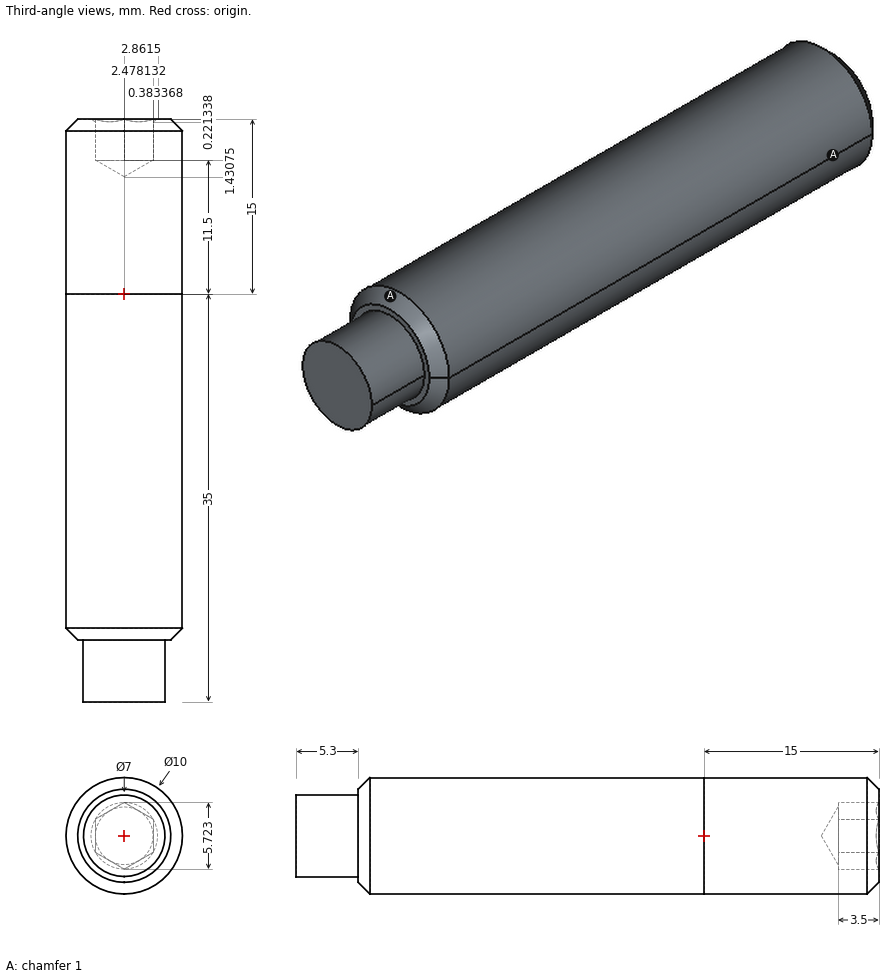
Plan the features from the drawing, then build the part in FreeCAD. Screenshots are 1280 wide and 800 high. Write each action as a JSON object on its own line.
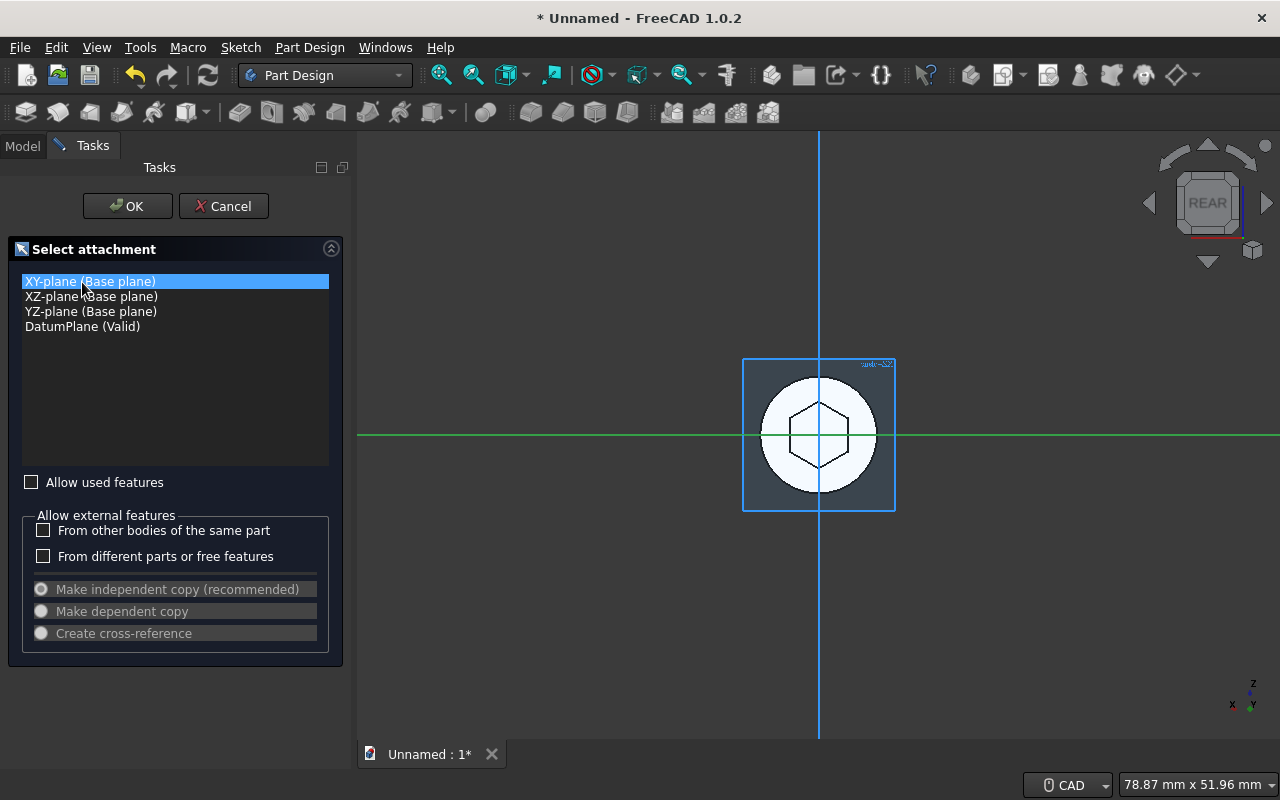
{"action": "left_click", "coordinate": [128, 206]}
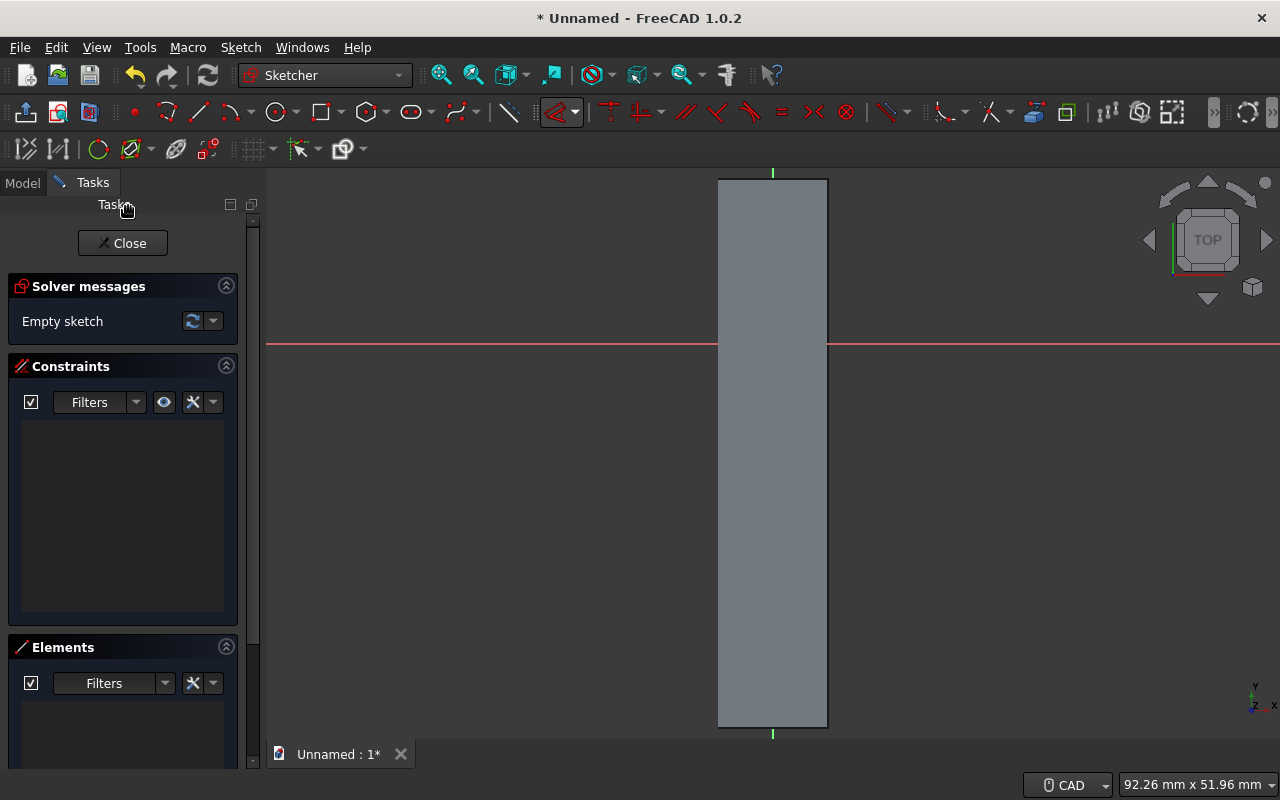
{"action": "left_click", "coordinate": [90, 112]}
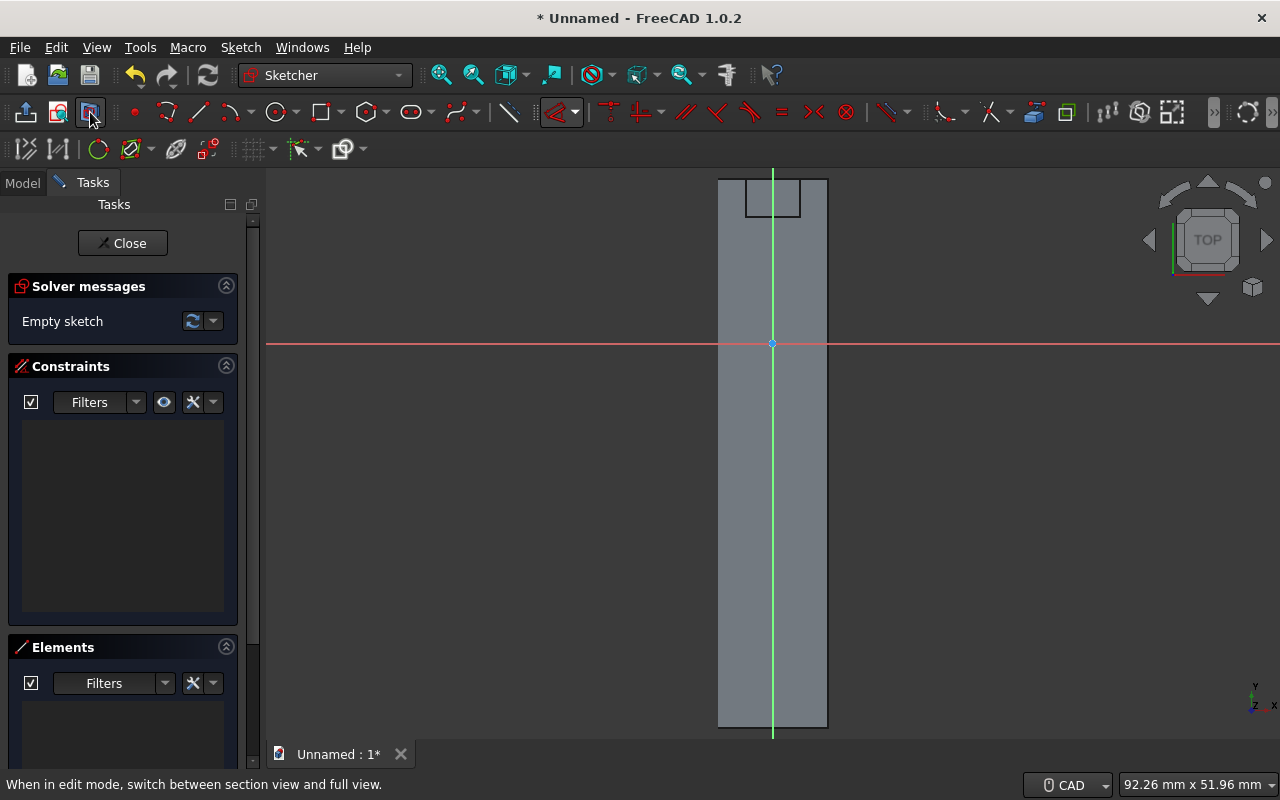
{"action": "scroll", "coordinate": [704, 454], "scroll_direction": "down", "scroll_amount": 5}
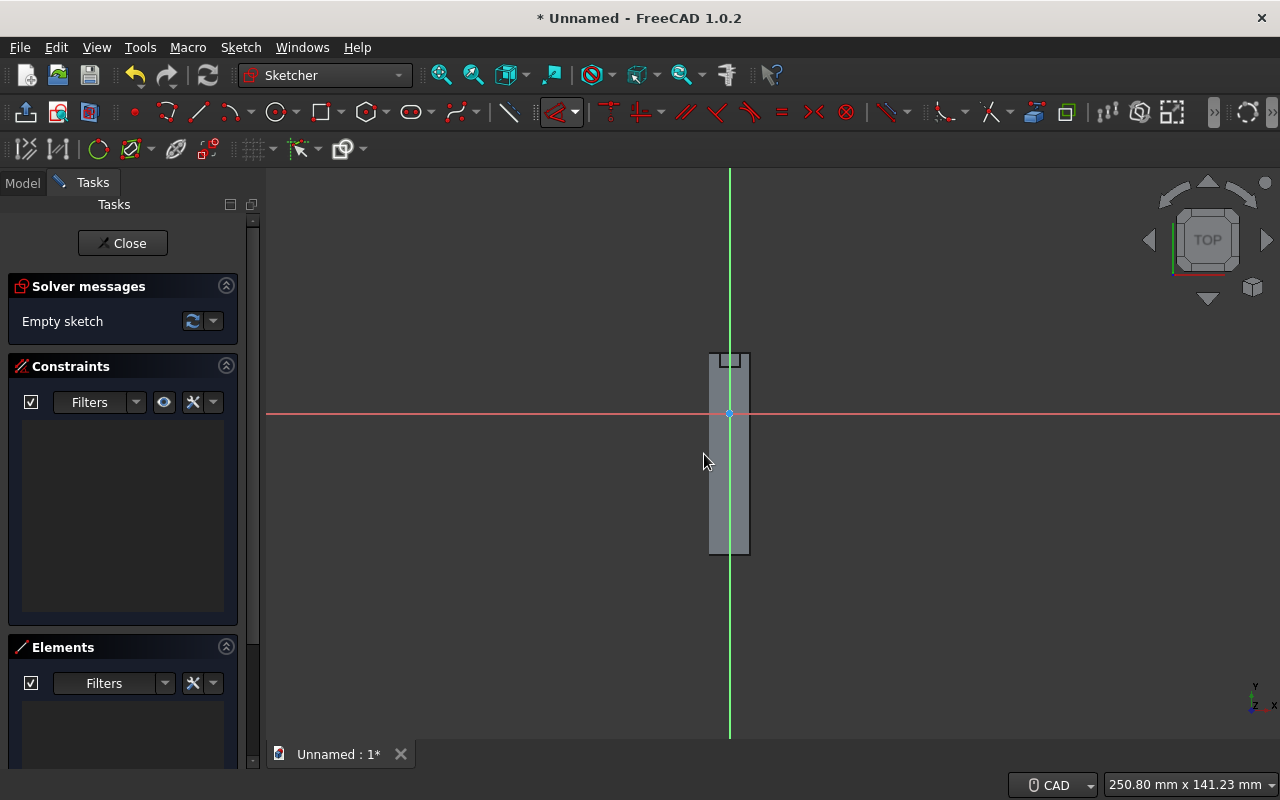
{"action": "scroll", "coordinate": [737, 358], "scroll_direction": "up", "scroll_amount": 15}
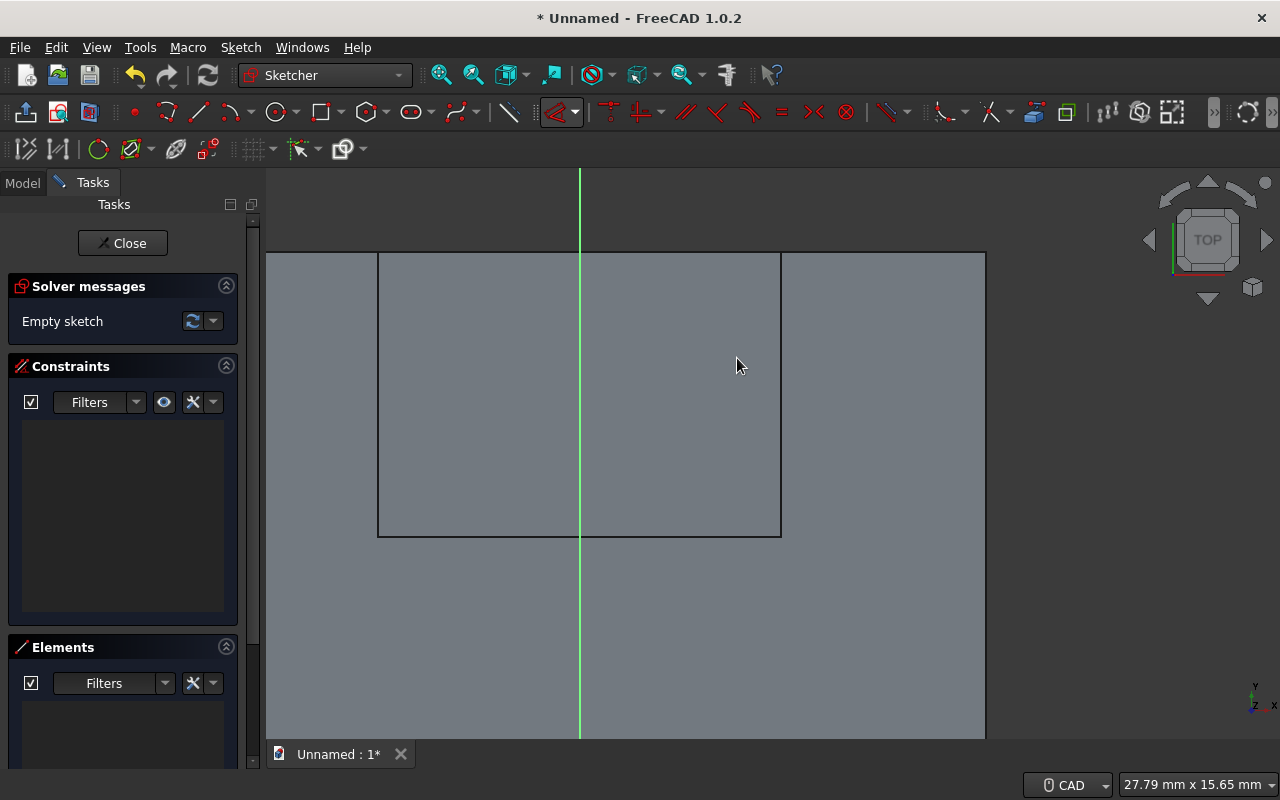
{"action": "left_click", "coordinate": [168, 112]}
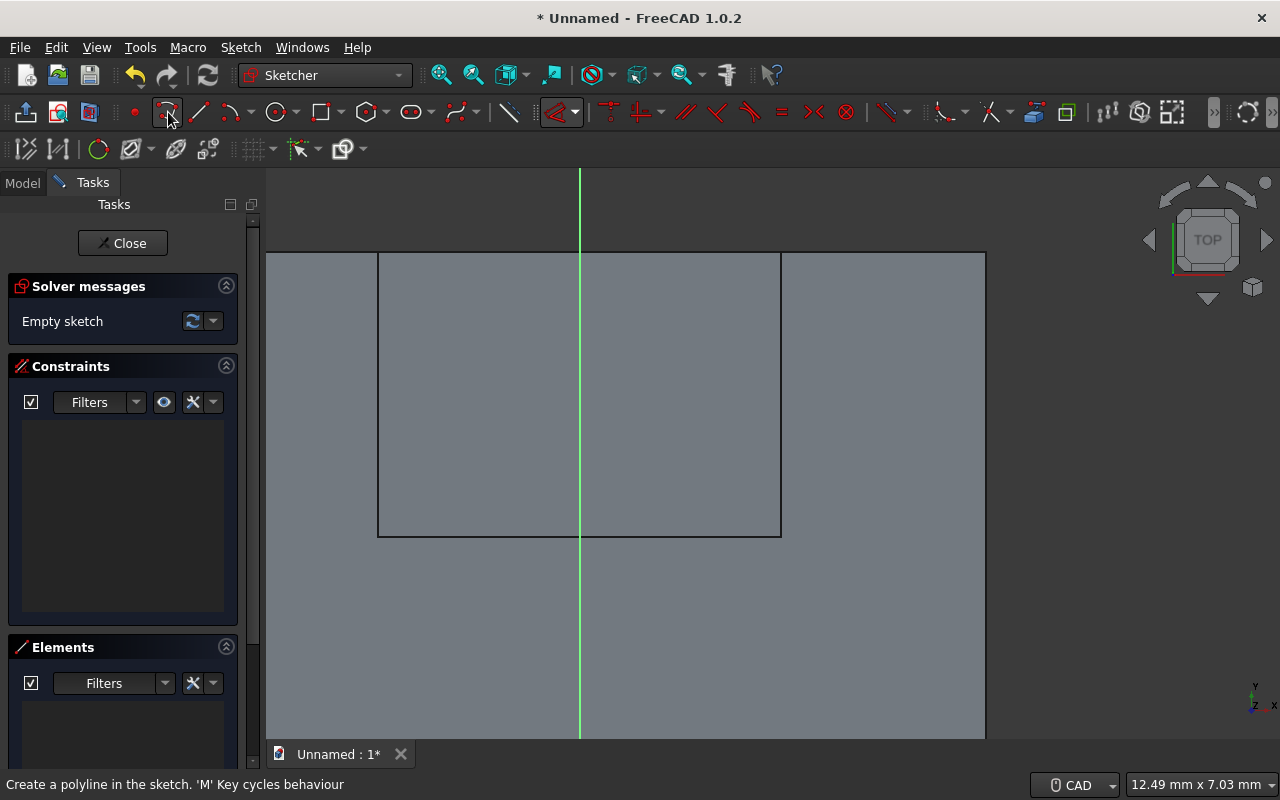
{"action": "left_click", "coordinate": [580, 653]}
{"action": "left_click", "coordinate": [781, 537]}
{"action": "left_click", "coordinate": [589, 537]}
{"action": "left_click", "coordinate": [580, 654]}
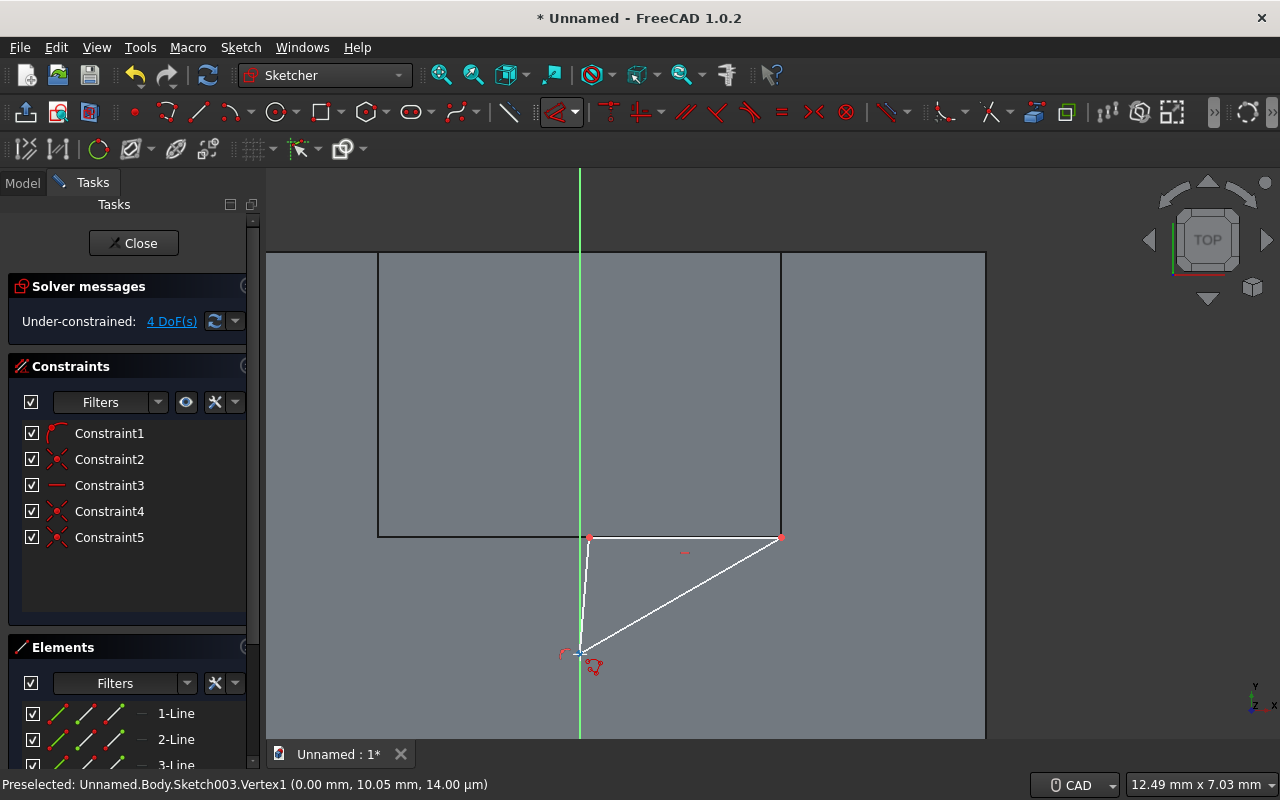
{"action": "left_click", "coordinate": [781, 270]}
{"action": "left_click", "coordinate": [812, 252]}
{"action": "left_click", "coordinate": [781, 252]}
{"action": "left_click", "coordinate": [781, 271]}
{"action": "key", "text": "Escape"}
{"action": "key", "text": "Escape"}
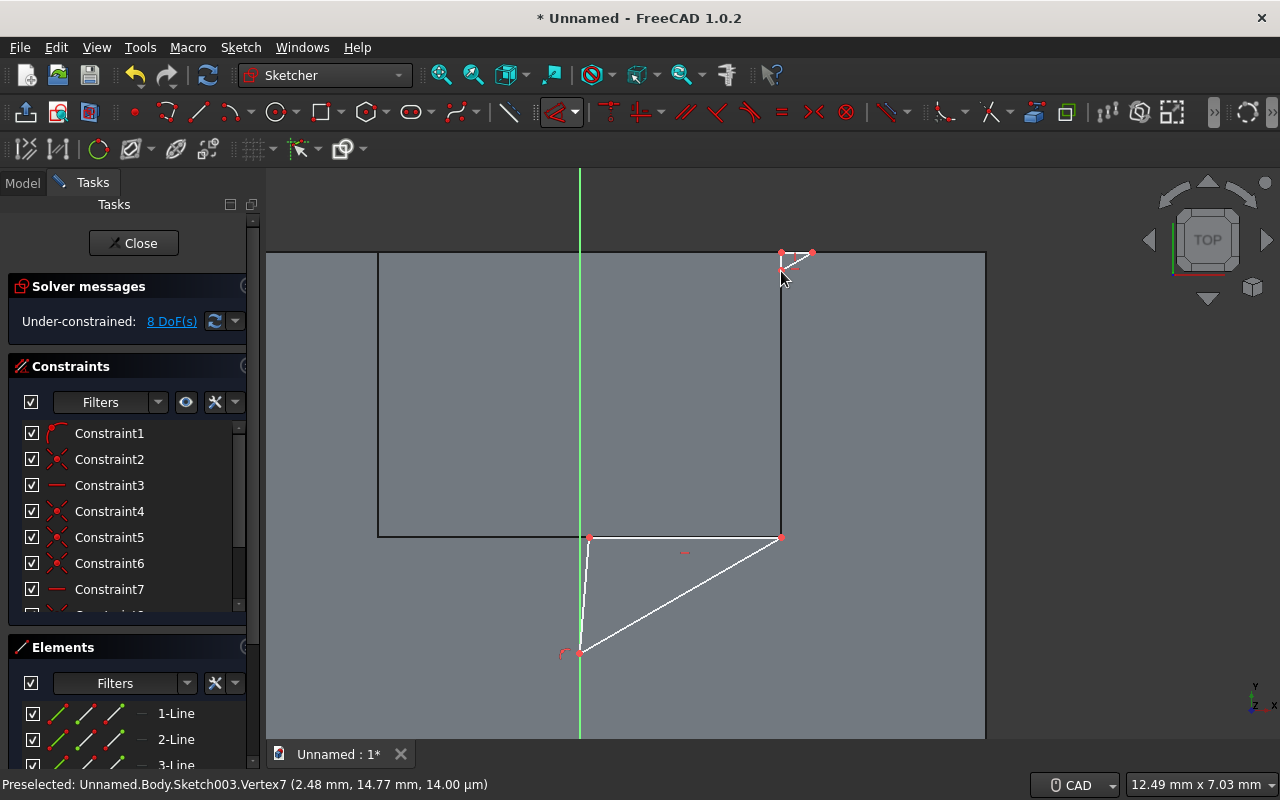
{"action": "left_click", "coordinate": [583, 619]}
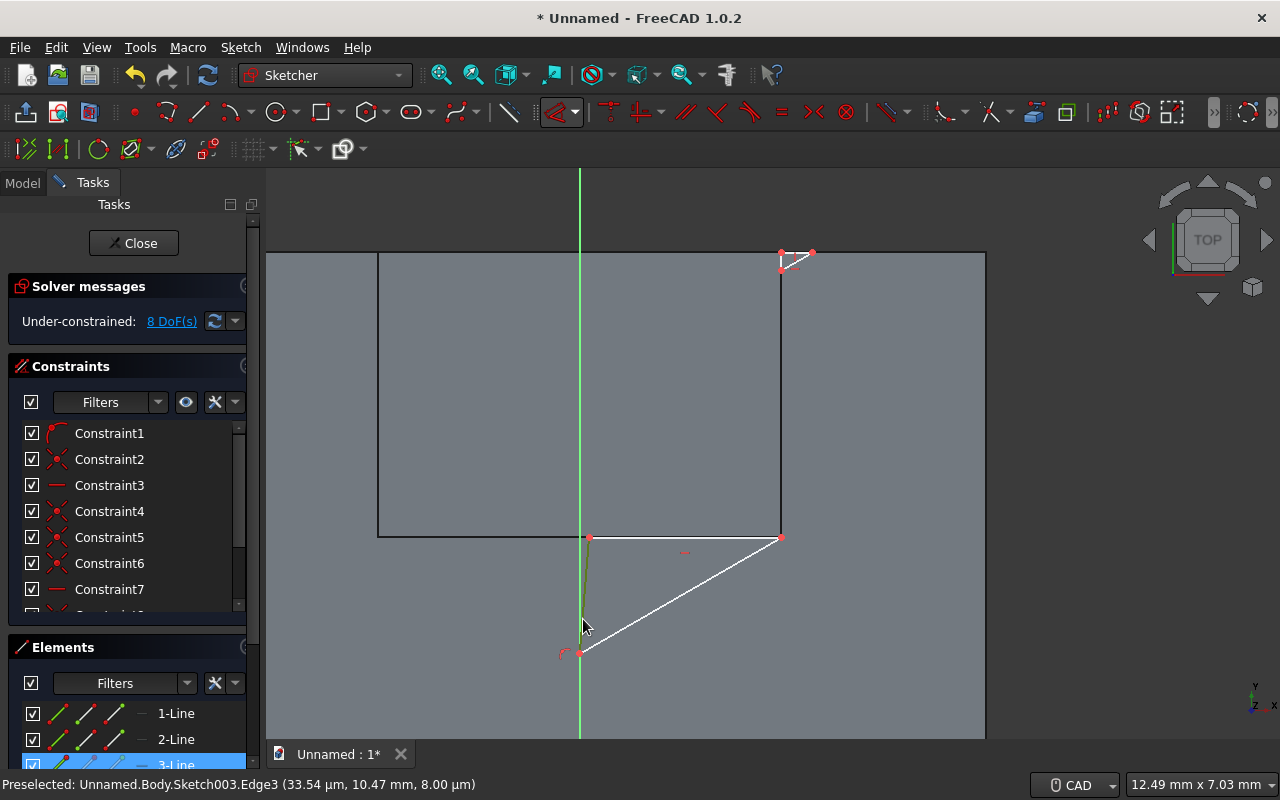
{"action": "key", "text": "v"}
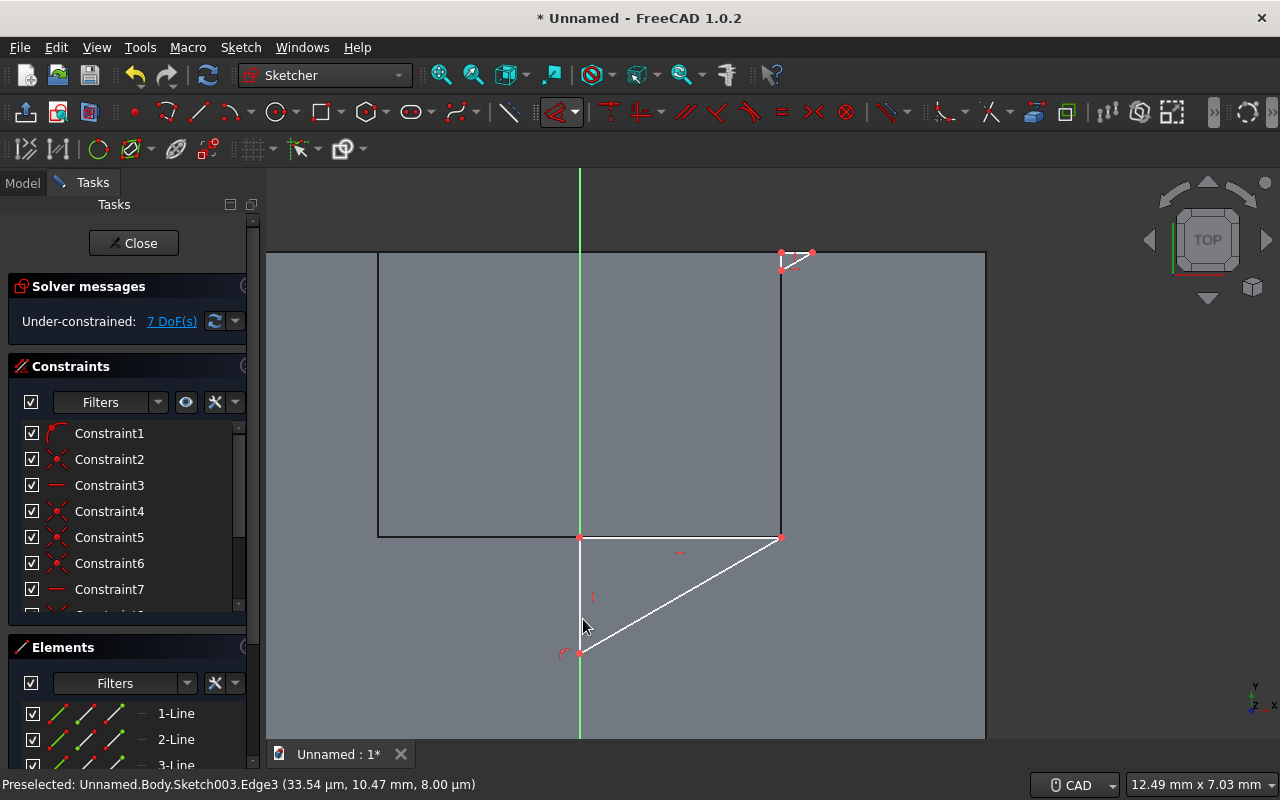
{"action": "left_click", "coordinate": [812, 253]}